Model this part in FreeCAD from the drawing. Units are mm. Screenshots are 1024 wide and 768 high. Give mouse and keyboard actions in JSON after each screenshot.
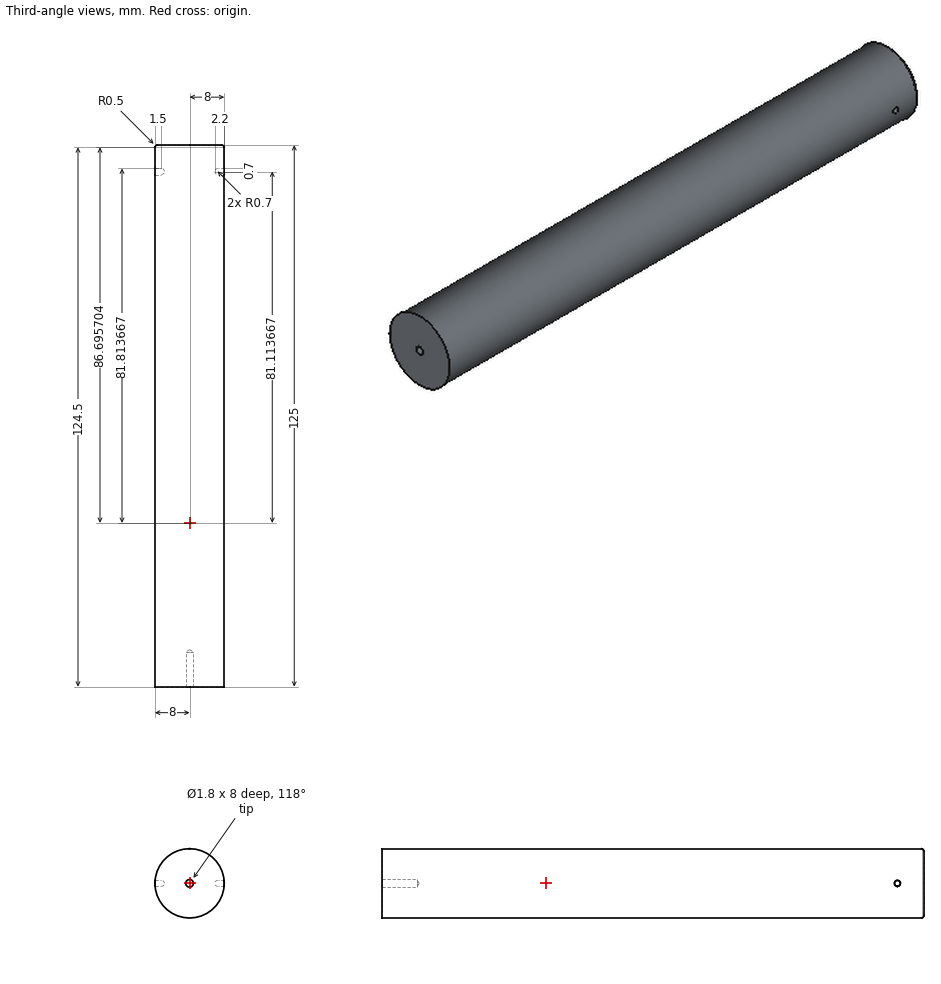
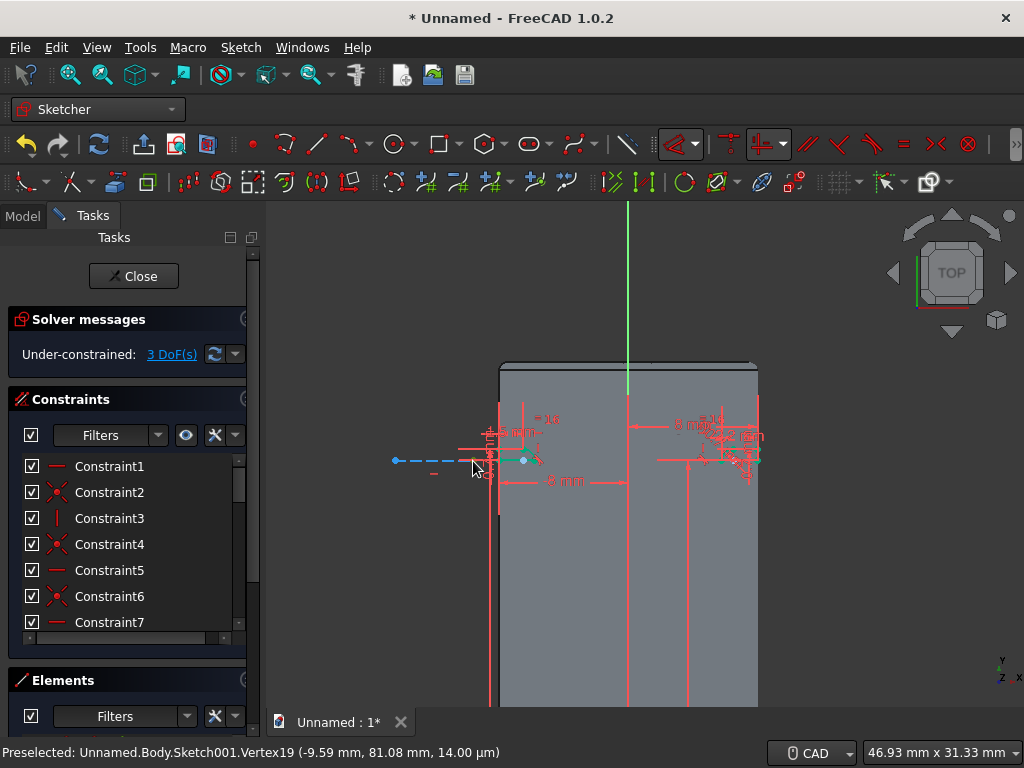
{"action": "key", "text": "i"}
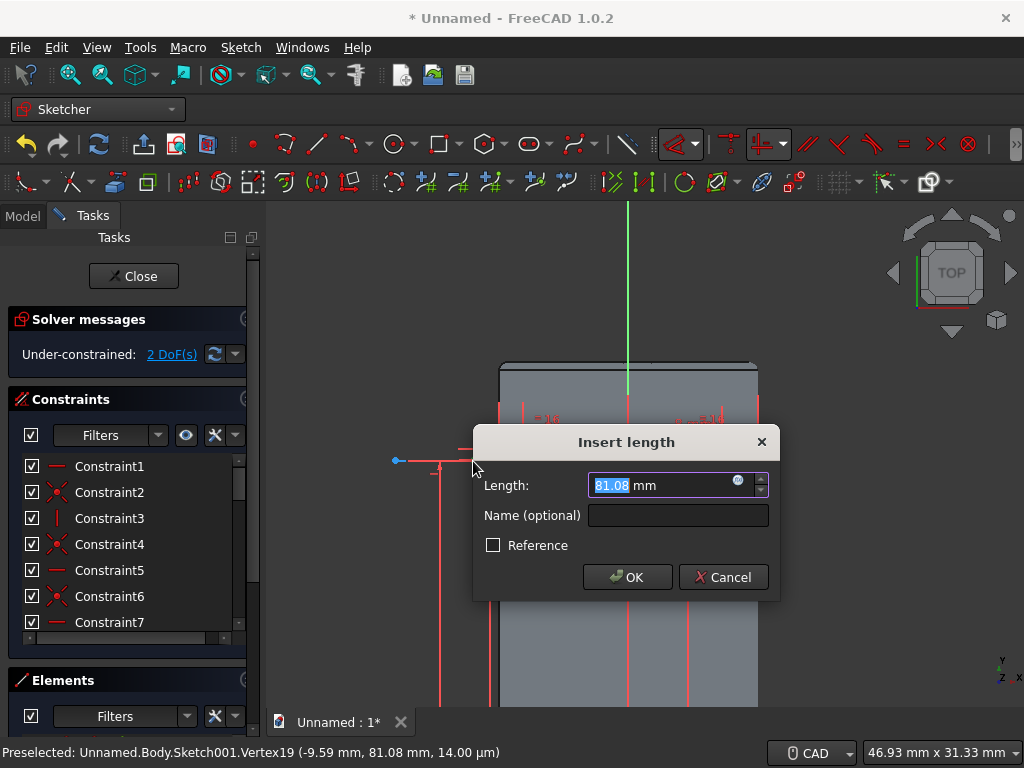
{"action": "type", "text": "81.113667"}
{"action": "key", "text": "Return"}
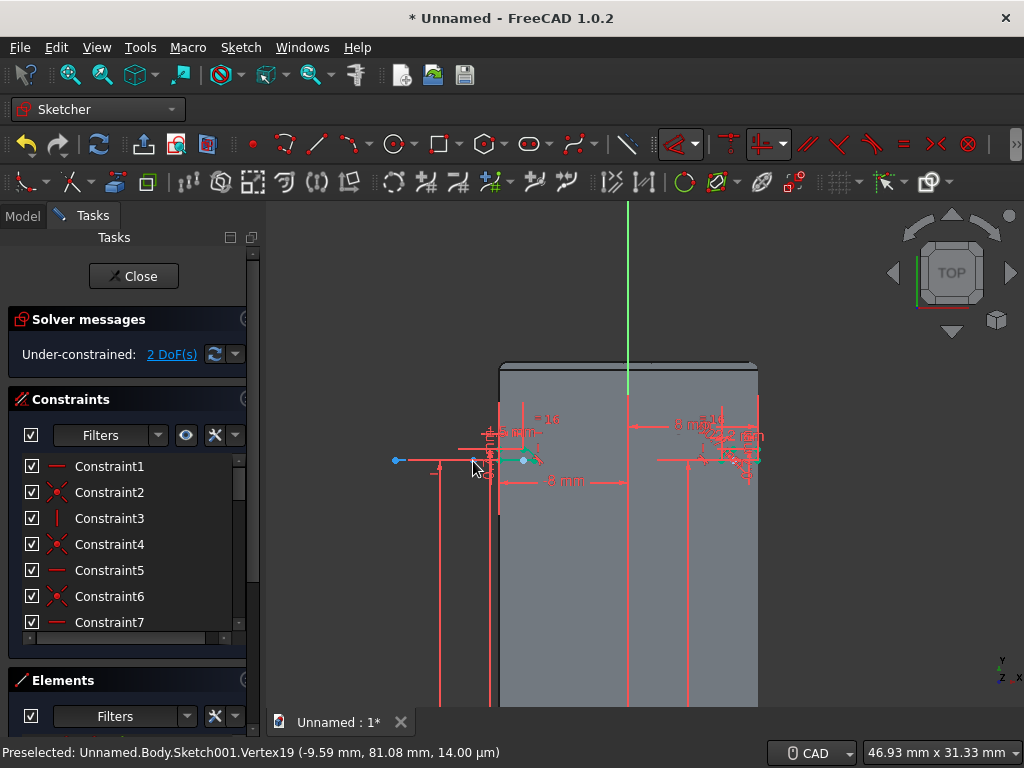
{"action": "left_click", "coordinate": [134, 276]}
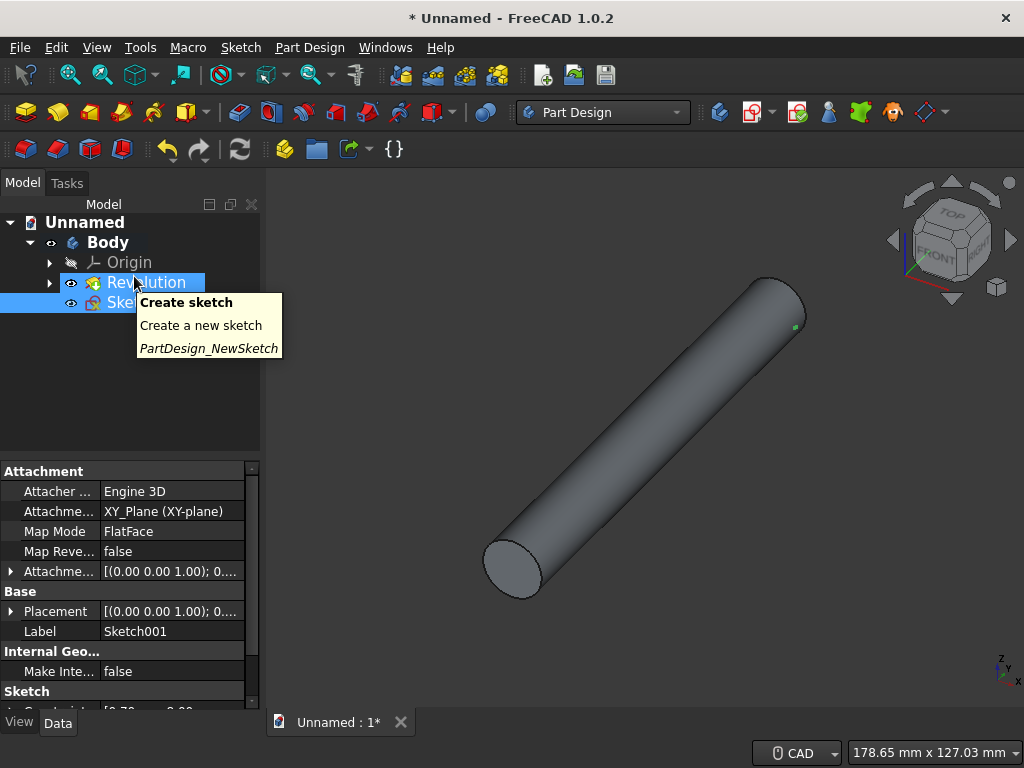
{"action": "left_click", "coordinate": [304, 112]}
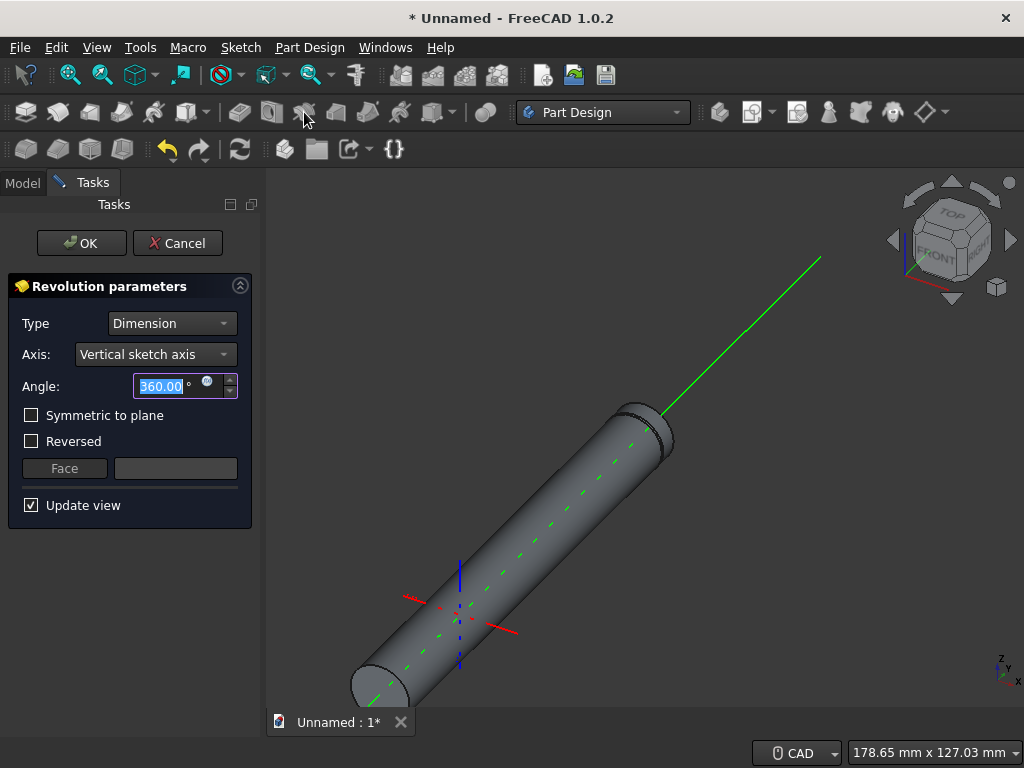
{"action": "left_click", "coordinate": [156, 354]}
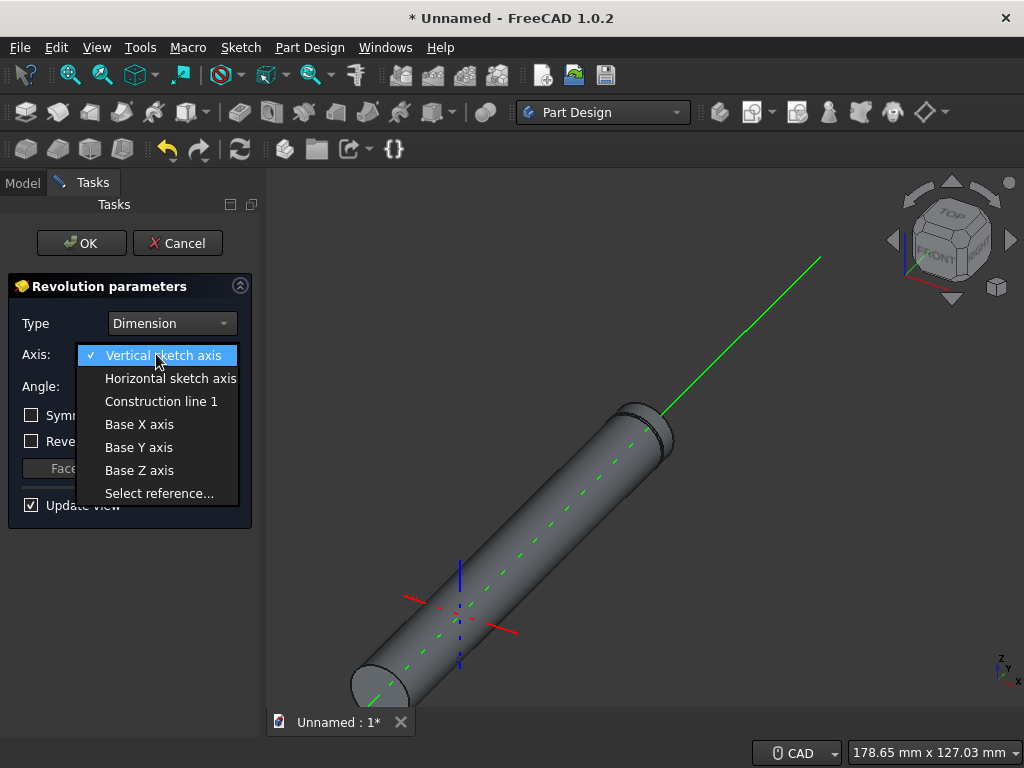
{"action": "left_click", "coordinate": [156, 402]}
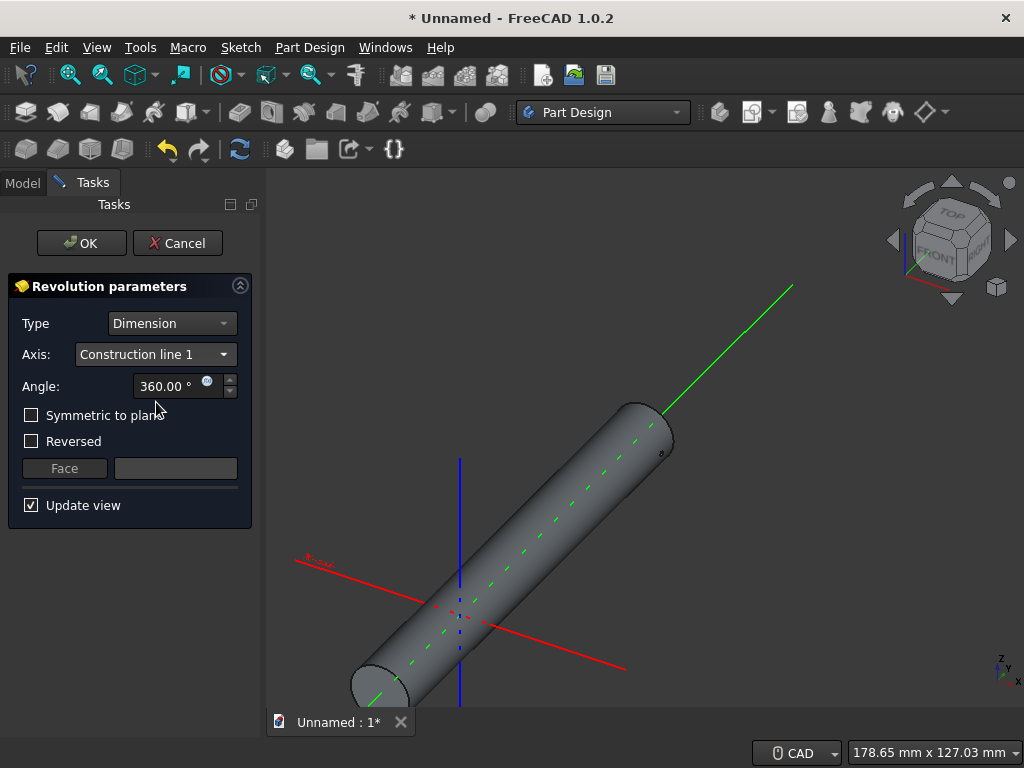
{"action": "left_click", "coordinate": [82, 243]}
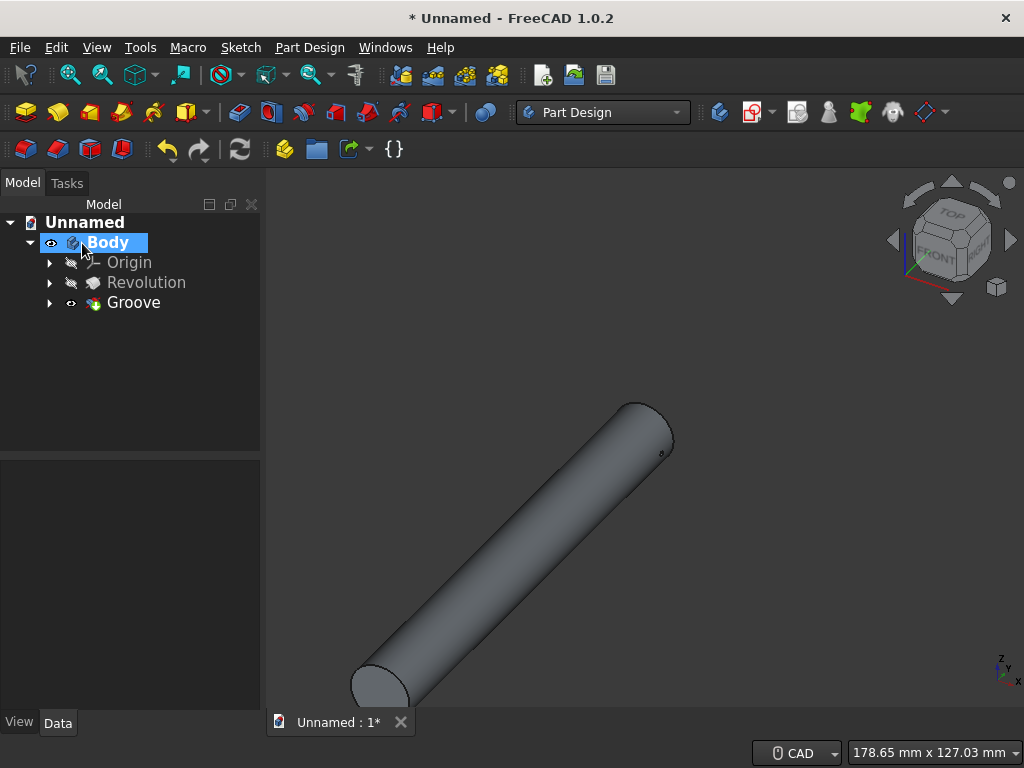
{"action": "left_click", "coordinate": [72, 76]}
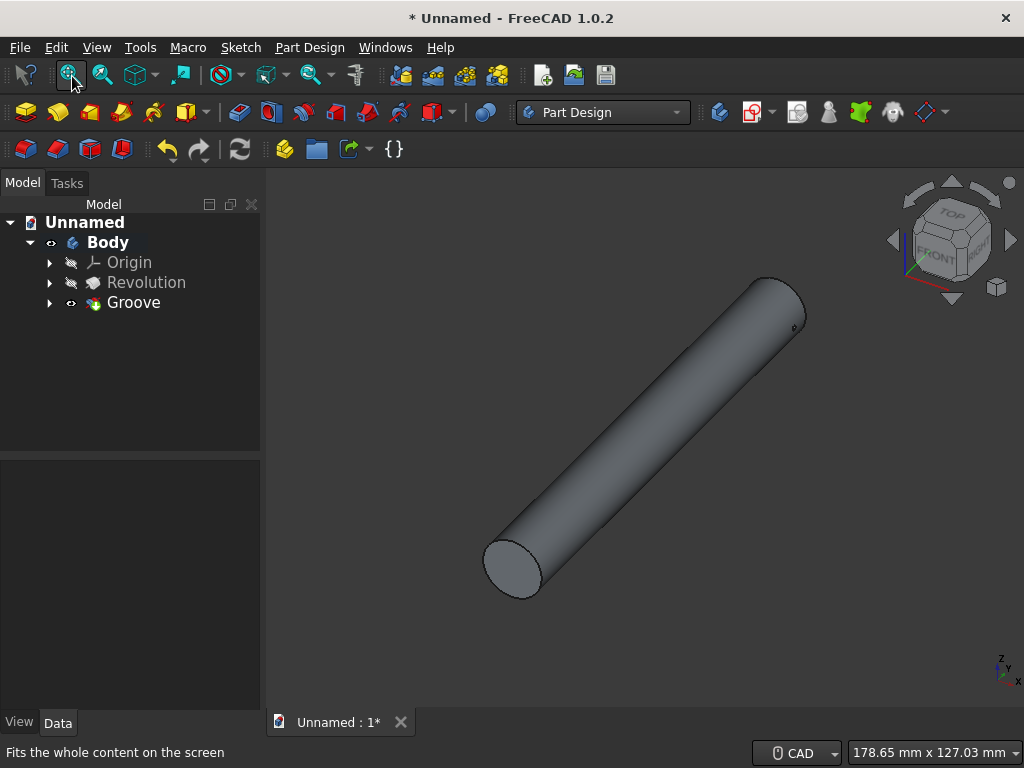
{"action": "left_click", "coordinate": [512, 568]}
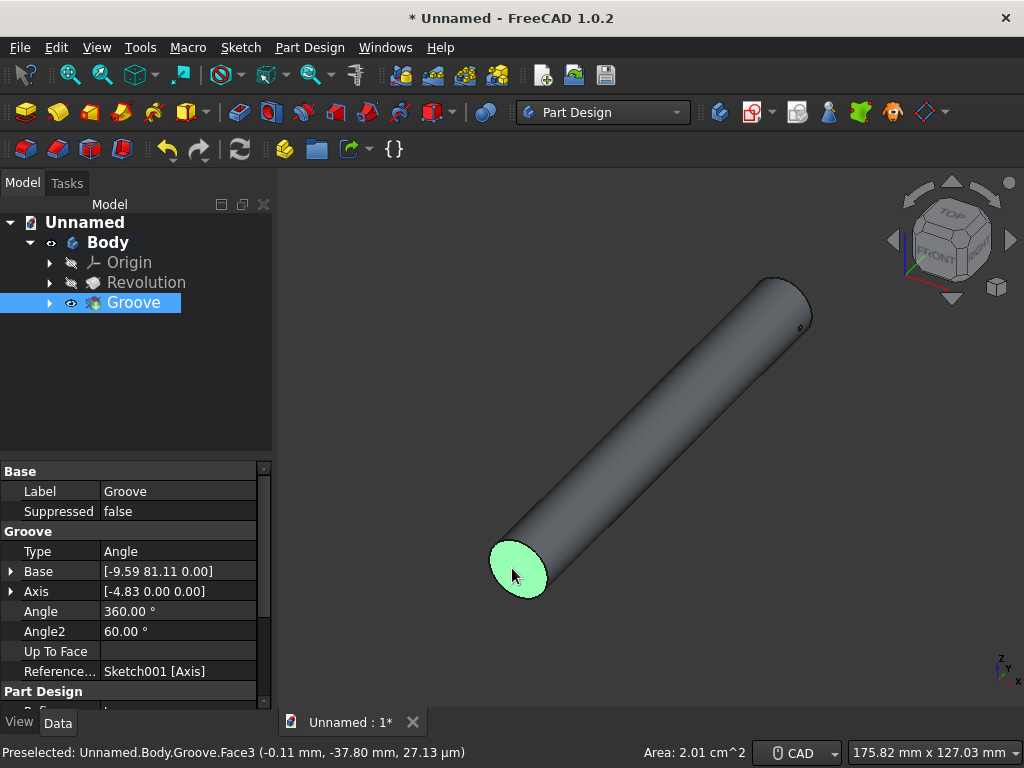
{"action": "left_click", "coordinate": [752, 112]}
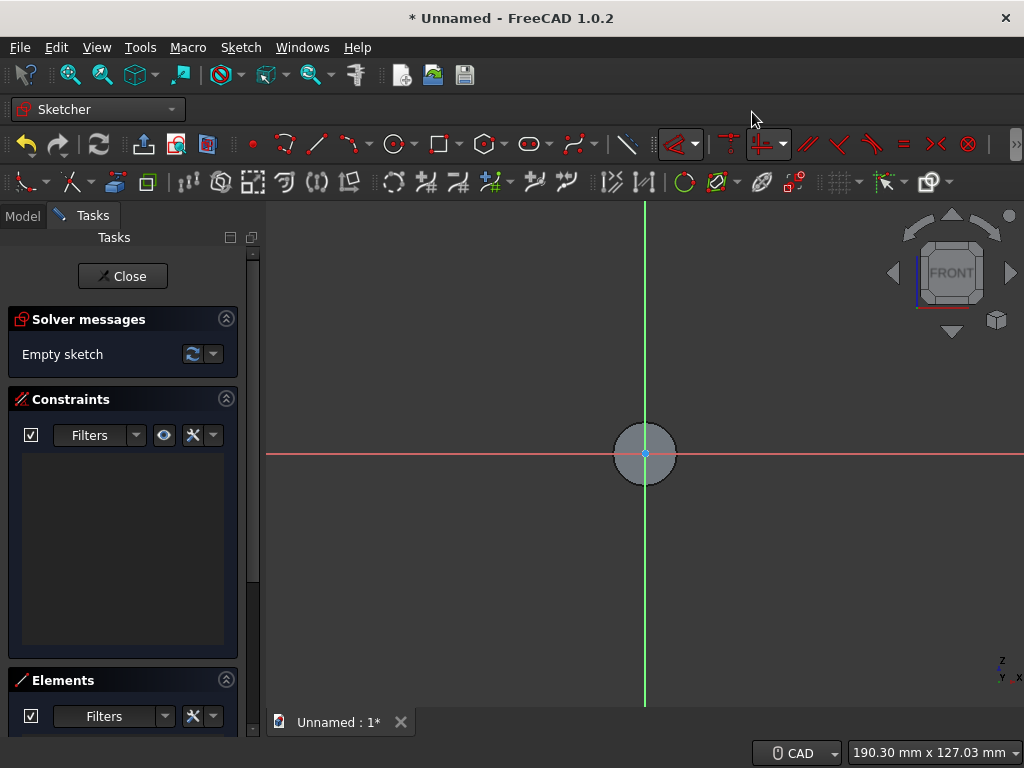
{"action": "scroll", "coordinate": [649, 454], "scroll_direction": "up", "scroll_amount": 15}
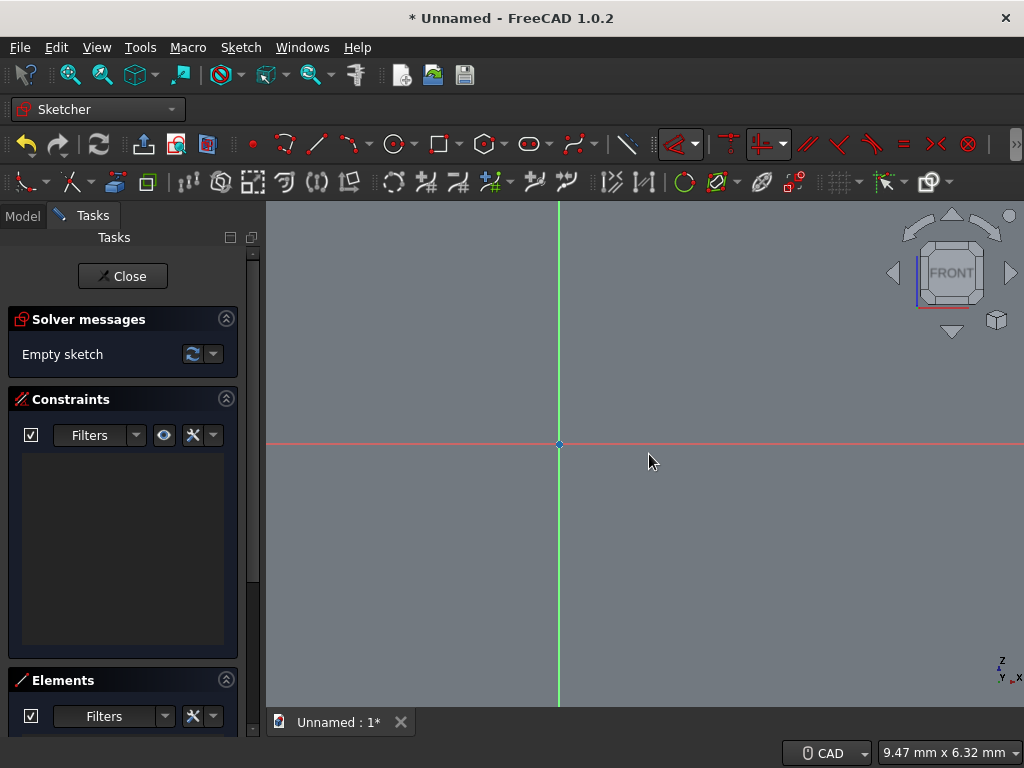
{"action": "scroll", "coordinate": [545, 437], "scroll_direction": "up", "scroll_amount": 4}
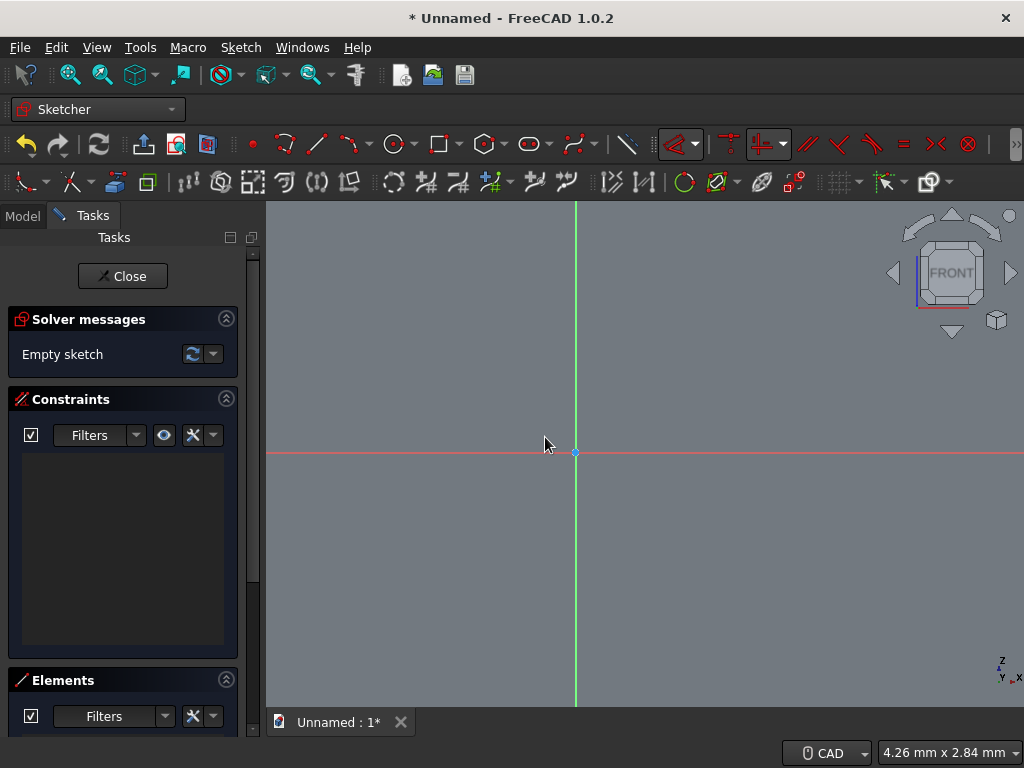
{"action": "key", "text": "g c"}